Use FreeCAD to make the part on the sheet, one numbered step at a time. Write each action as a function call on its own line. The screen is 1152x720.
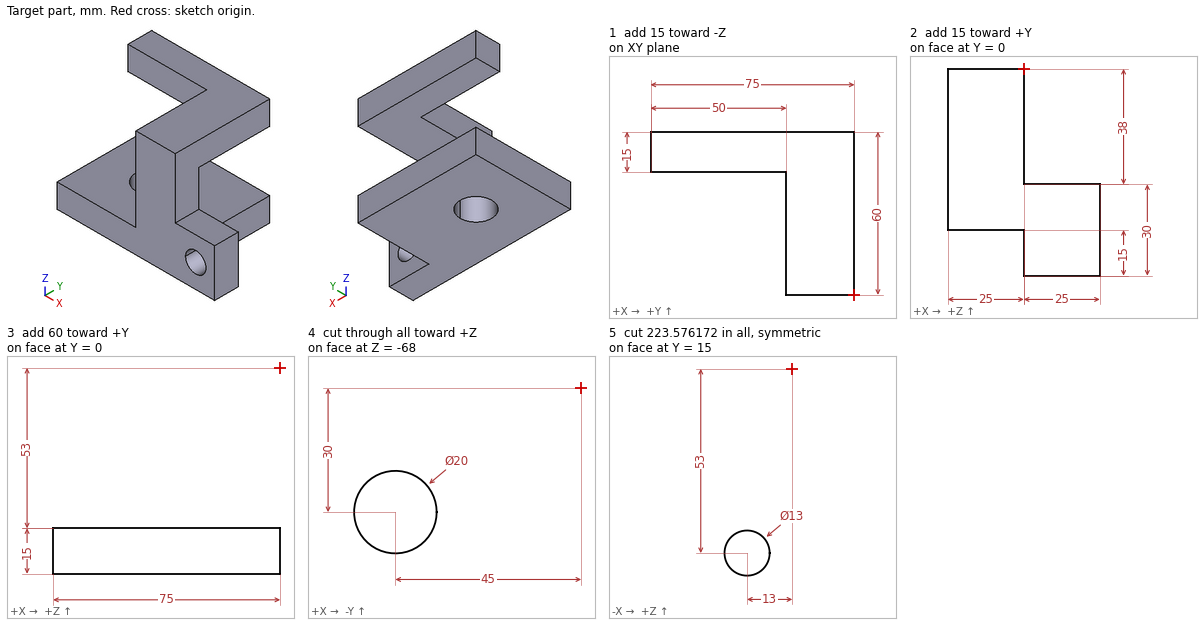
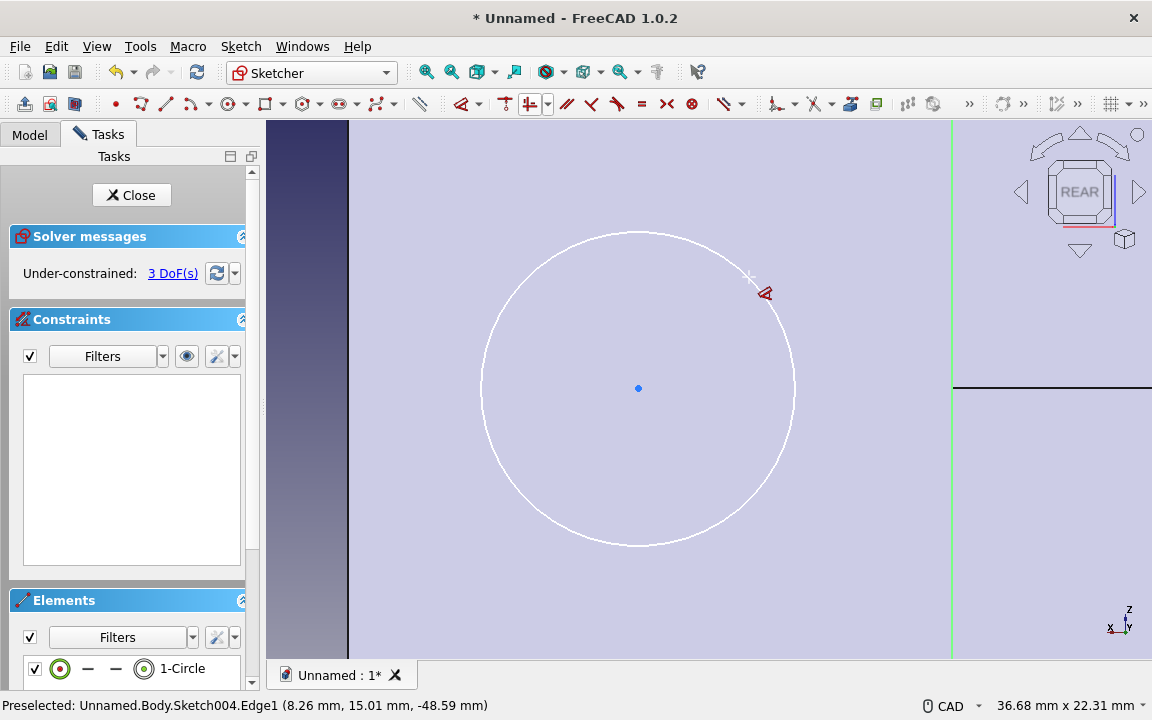
click(749, 278)
click(772, 255)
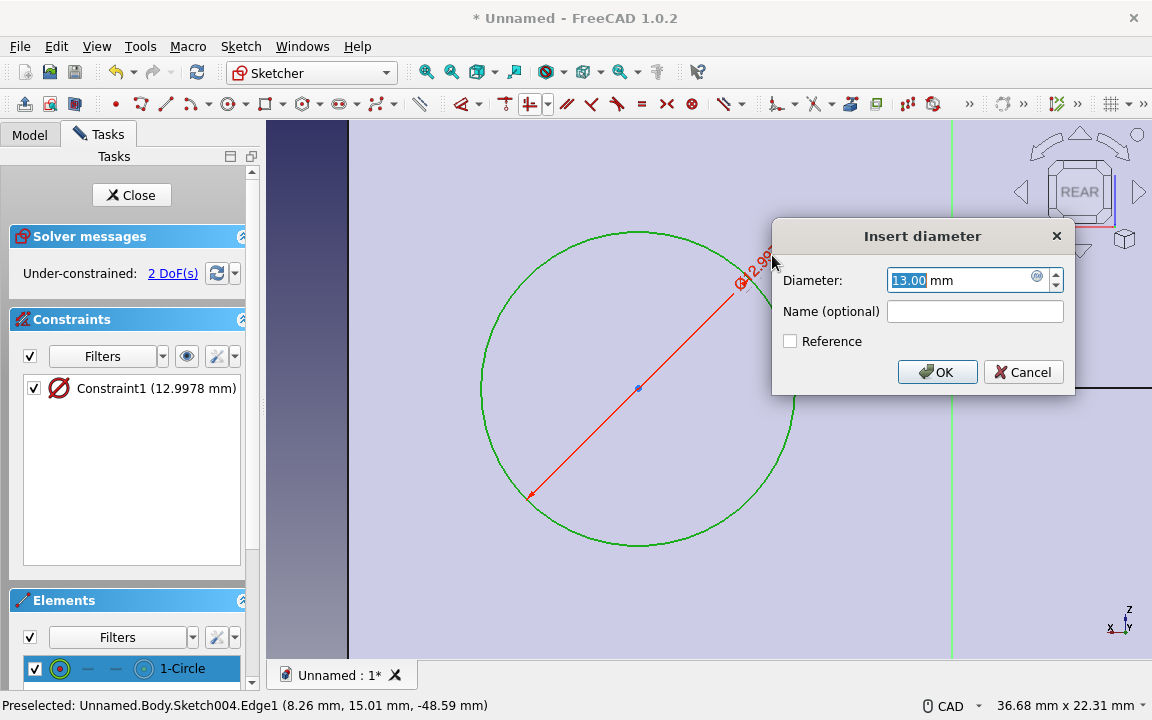
text(13)
key(Return)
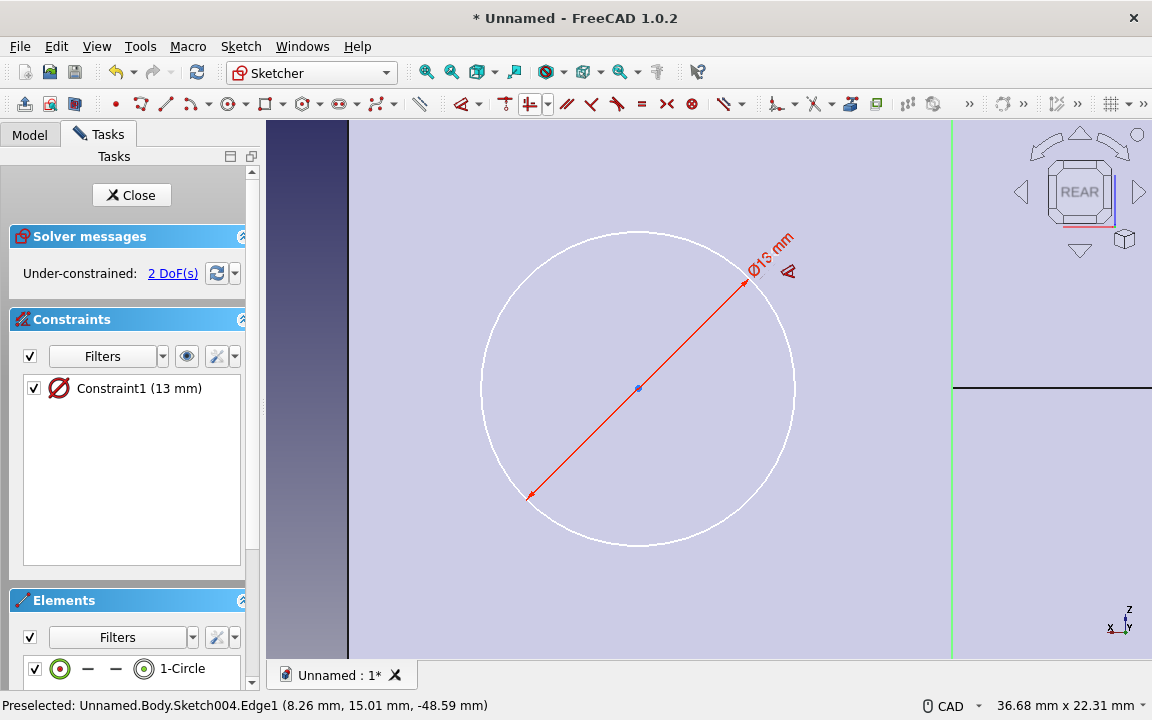
click(638, 389)
click(723, 423)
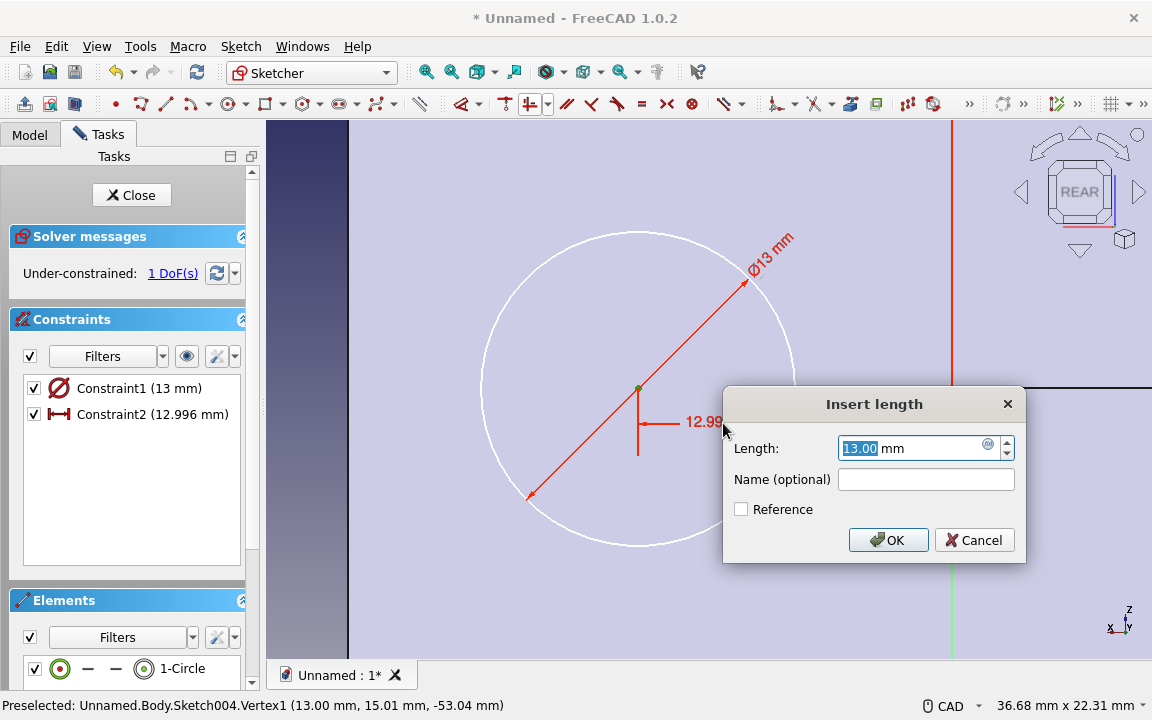
text(13)
key(Return)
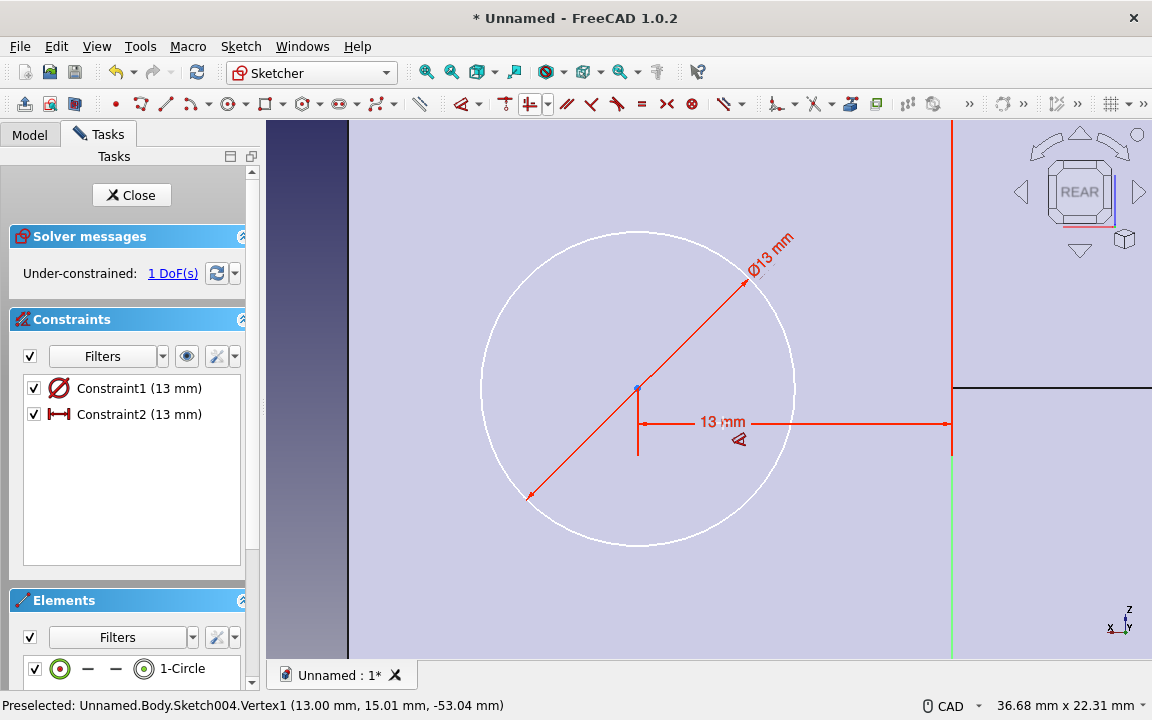
click(638, 389)
click(986, 269)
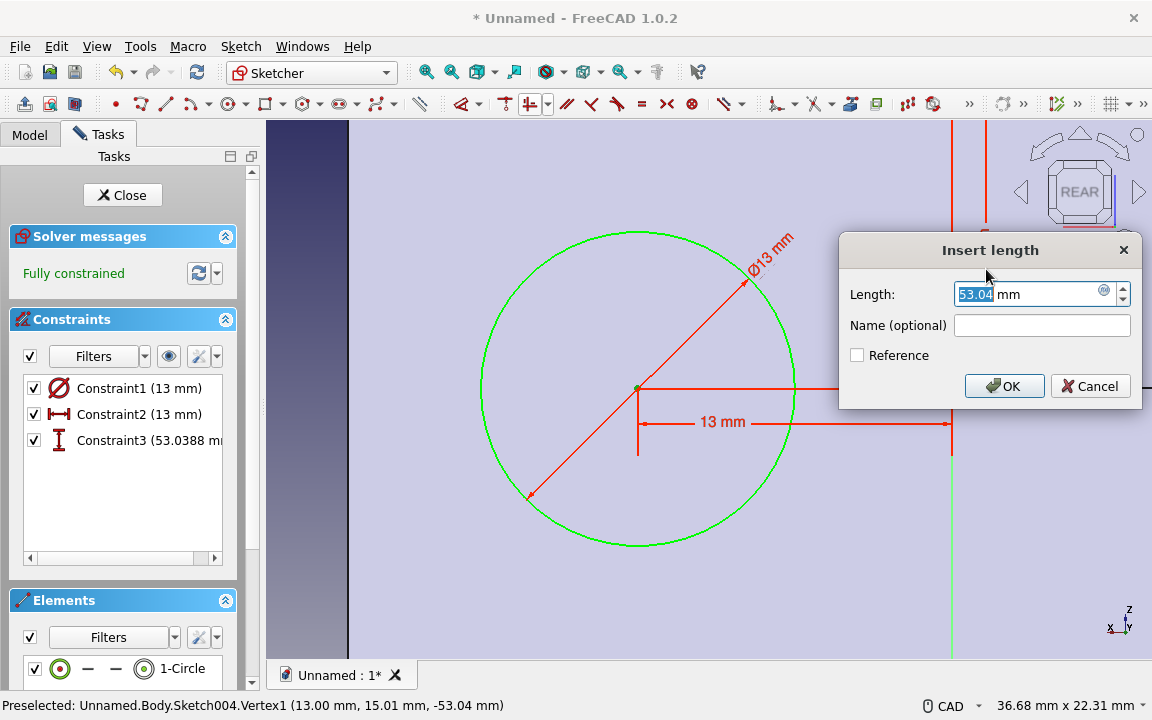
text(53)
key(Return)
key(Escape)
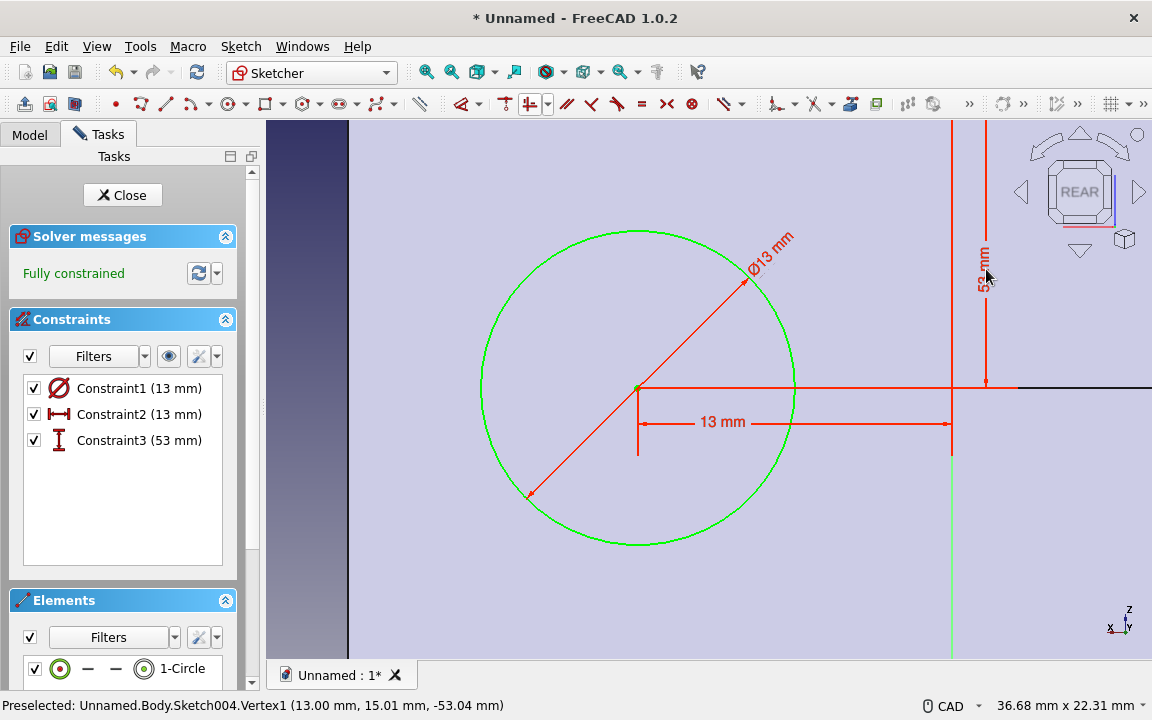
click(123, 195)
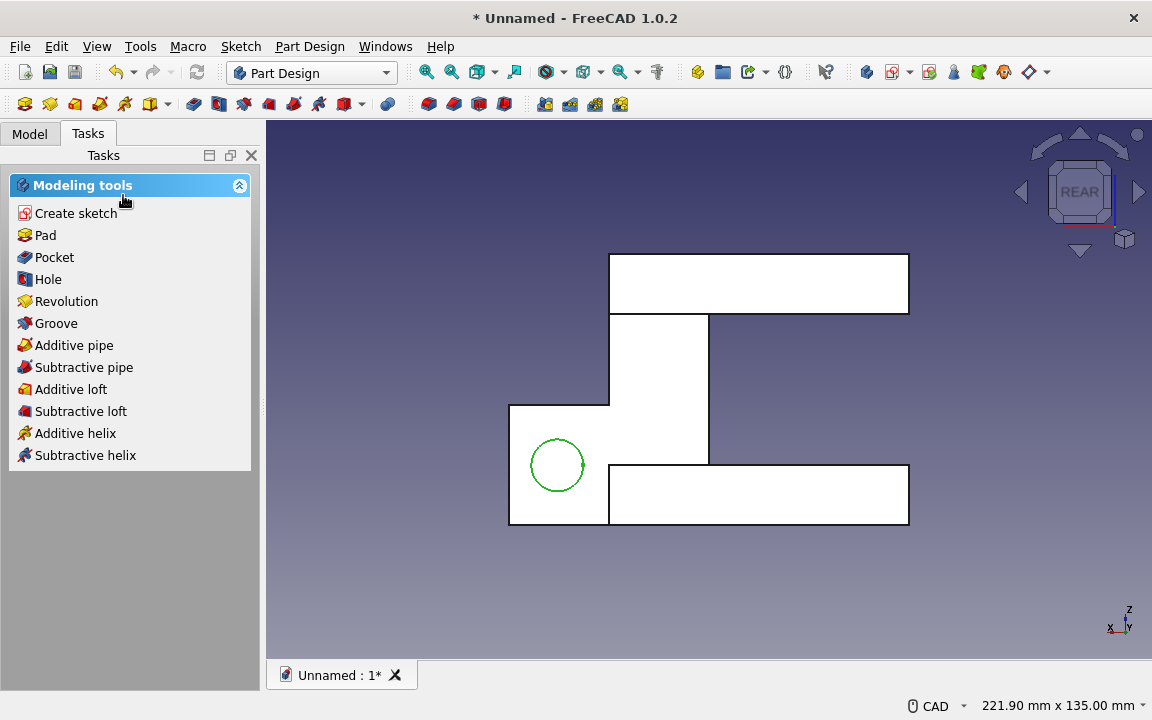
click(194, 104)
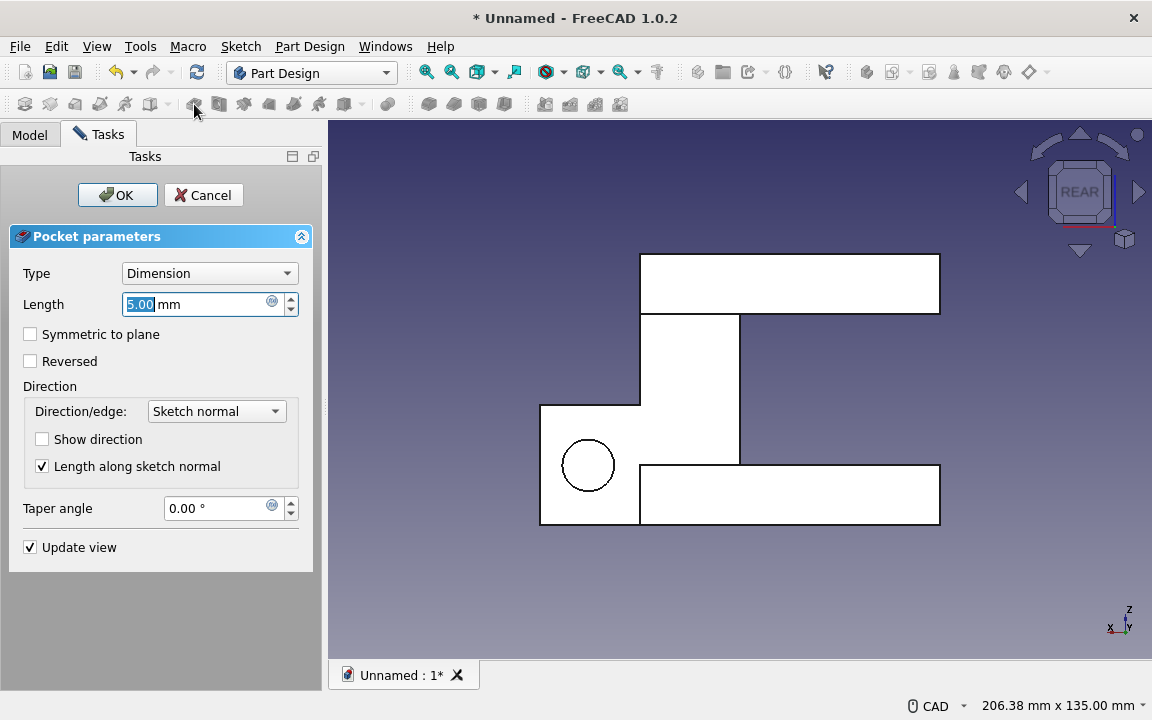
text(223.576172)
key(Tab)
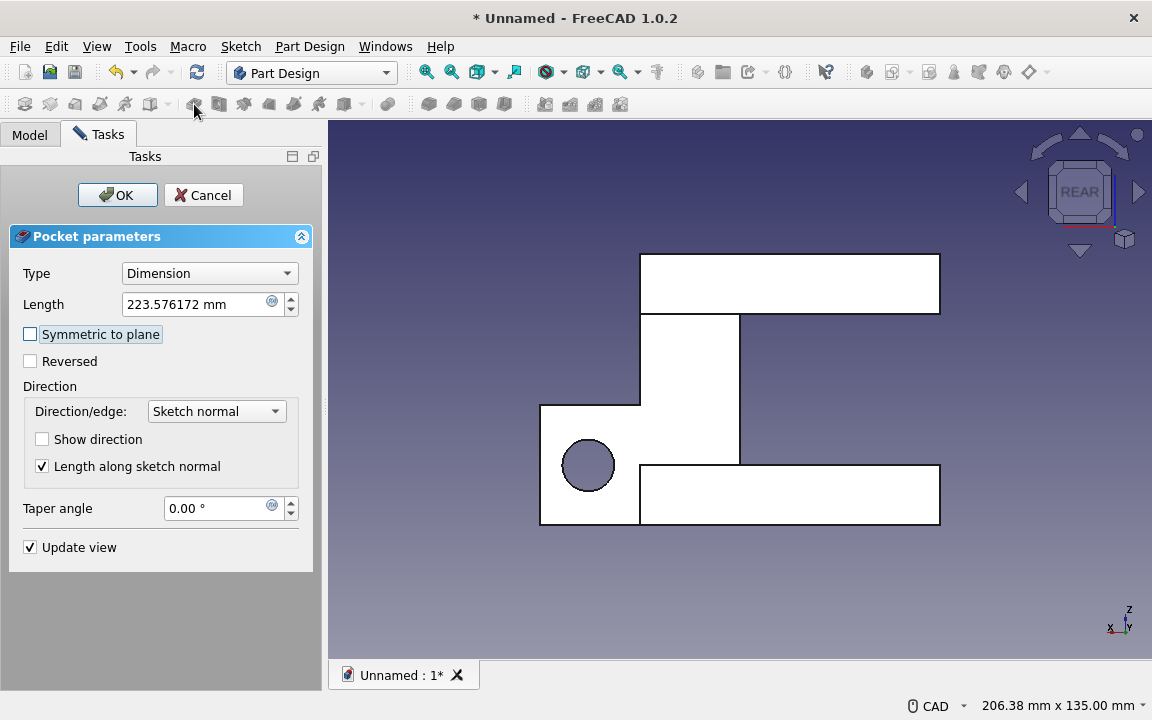
click(31, 334)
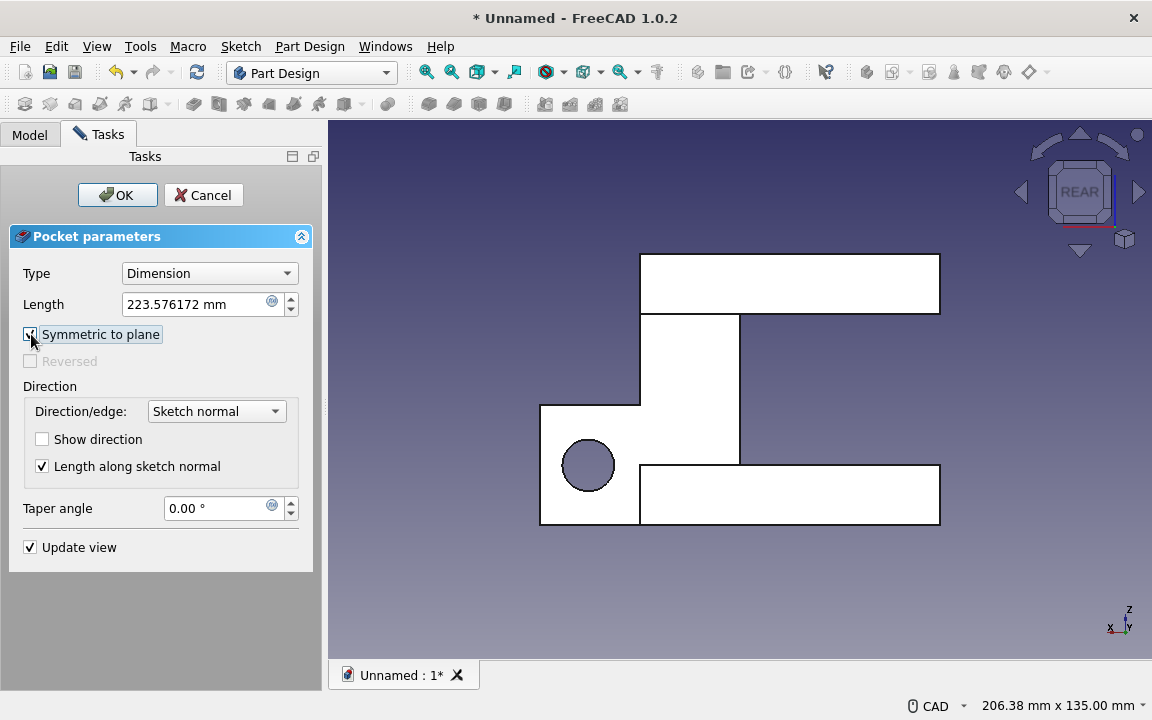
click(118, 195)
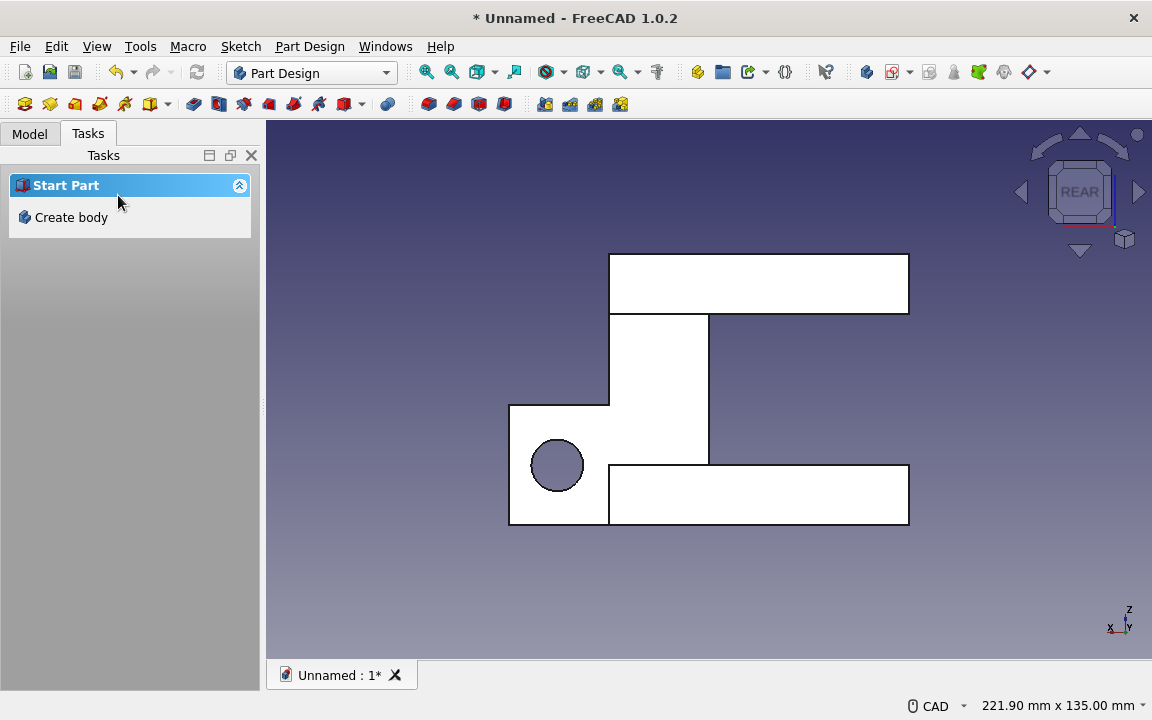
key(0)